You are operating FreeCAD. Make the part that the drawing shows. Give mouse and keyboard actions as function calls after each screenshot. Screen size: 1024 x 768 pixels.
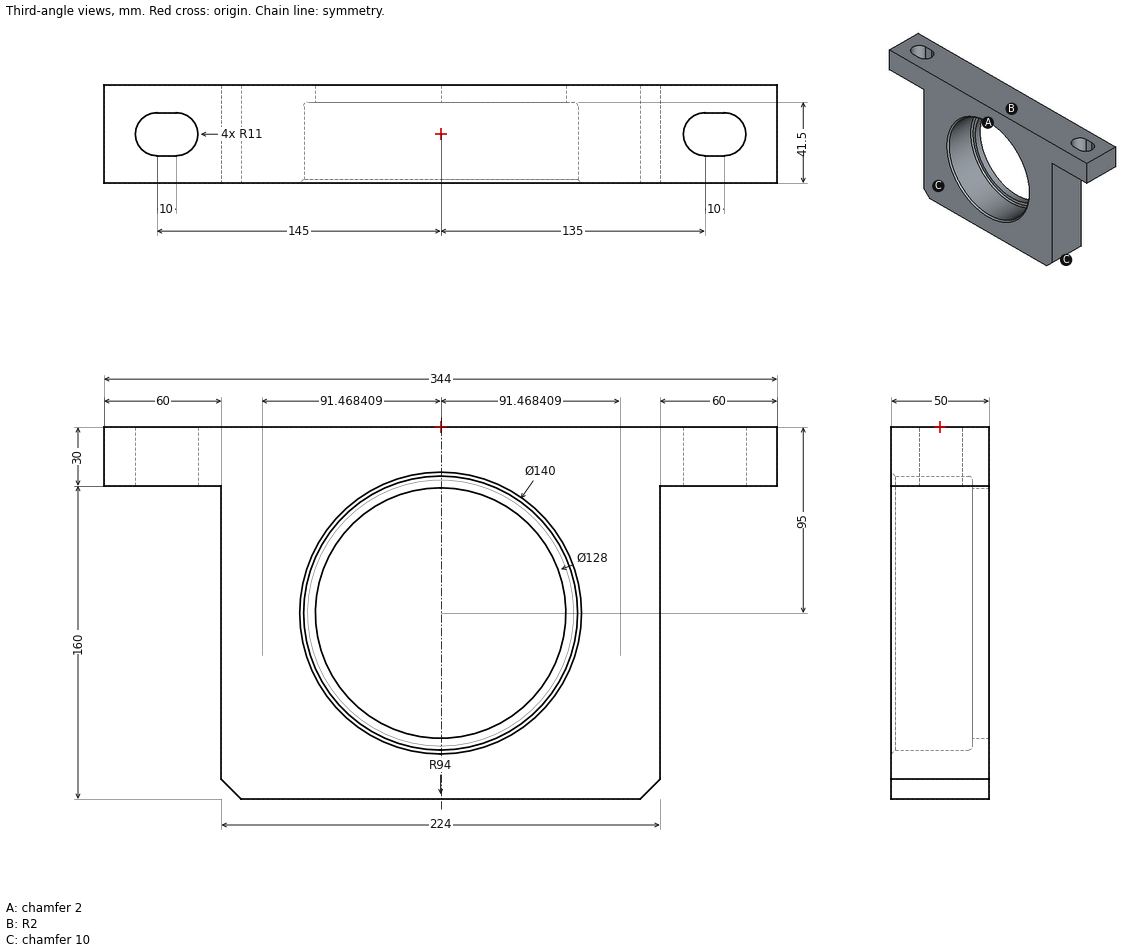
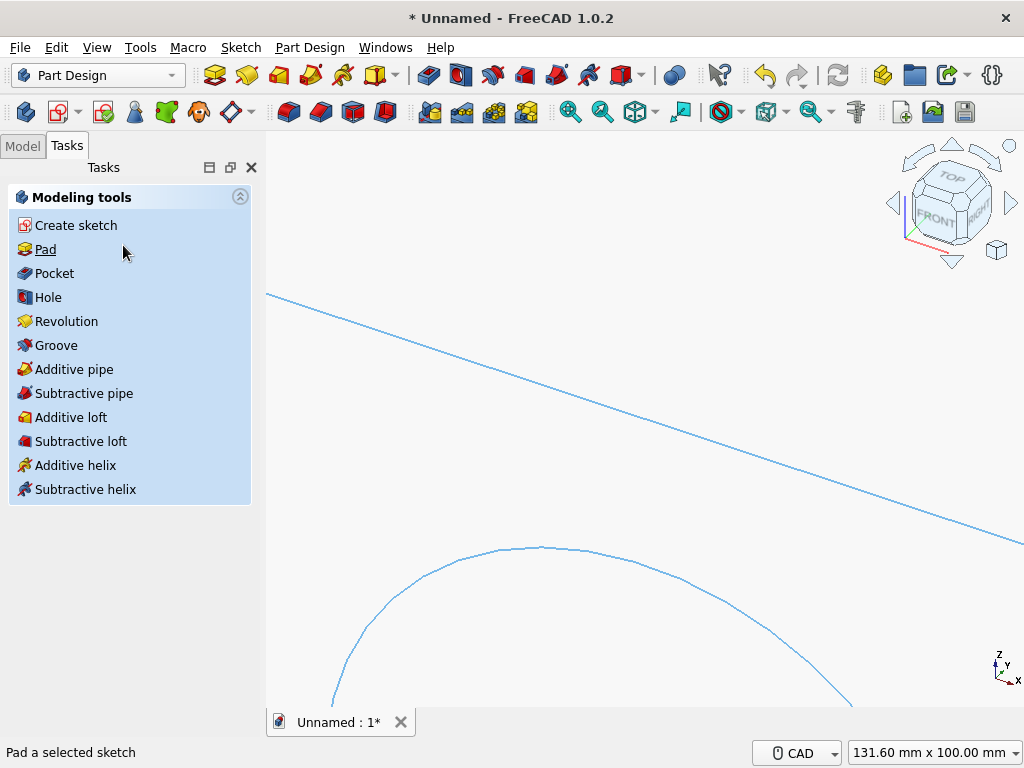
click(216, 76)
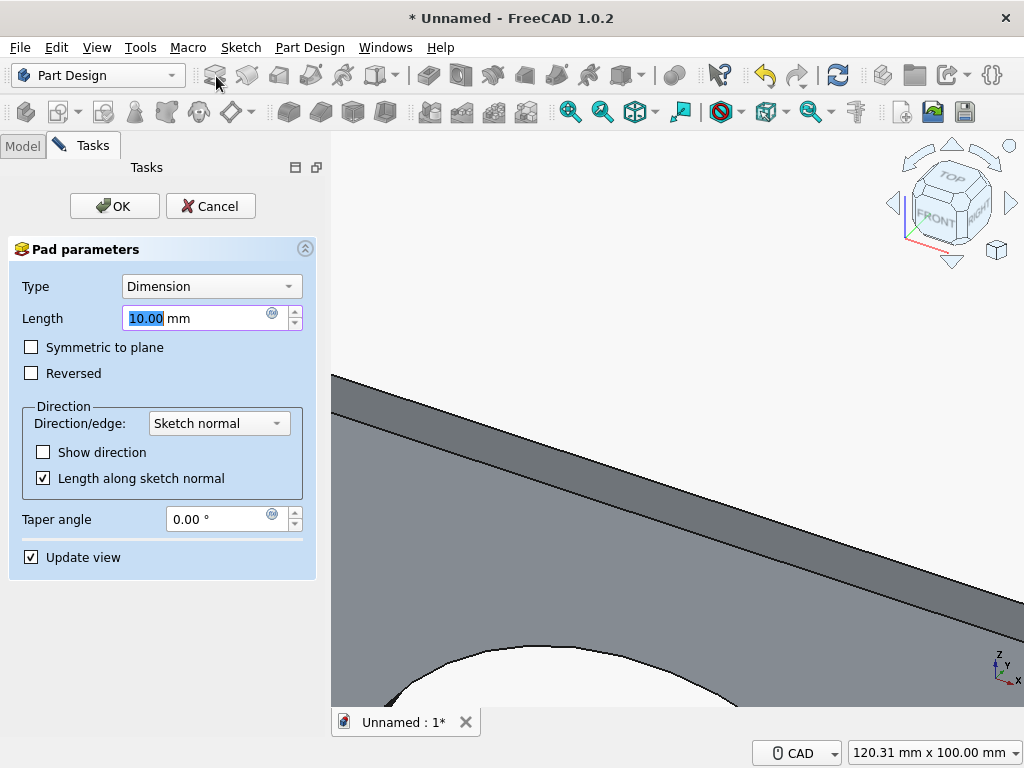
text(50)
key(Tab)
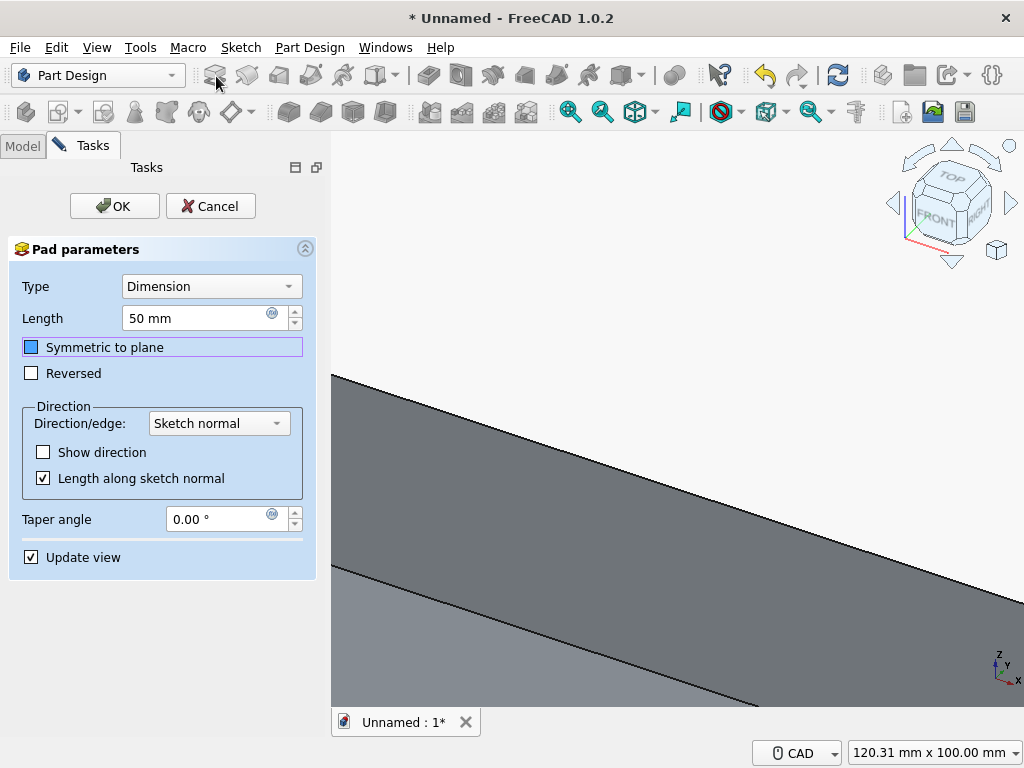
click(30, 347)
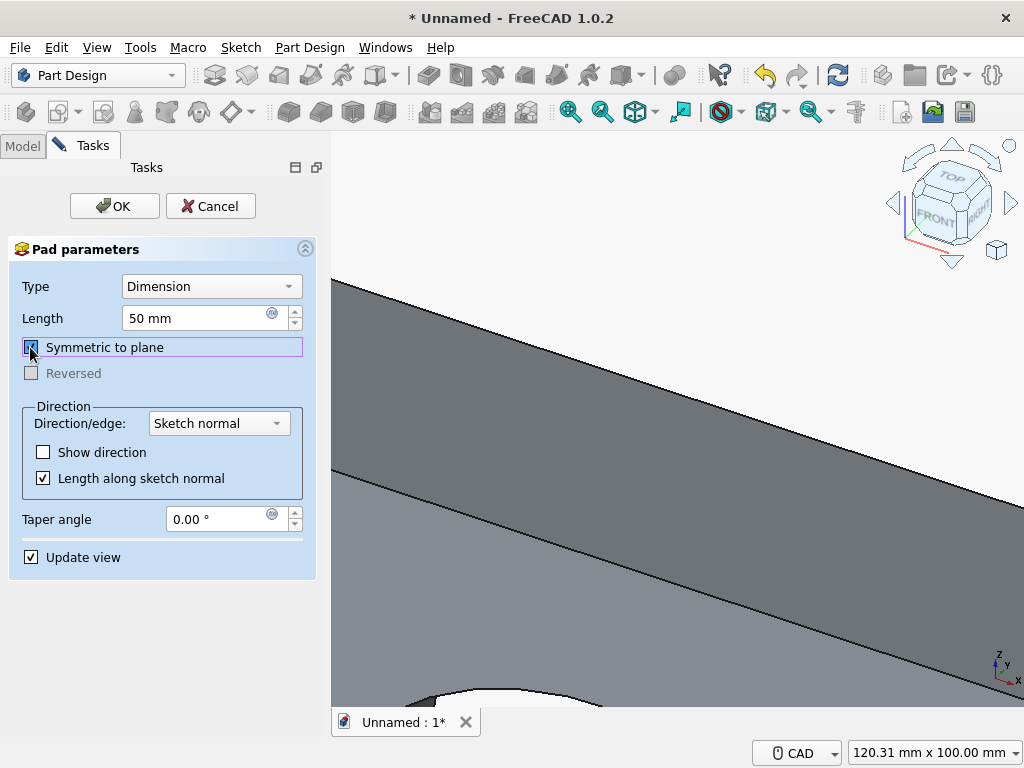
click(115, 206)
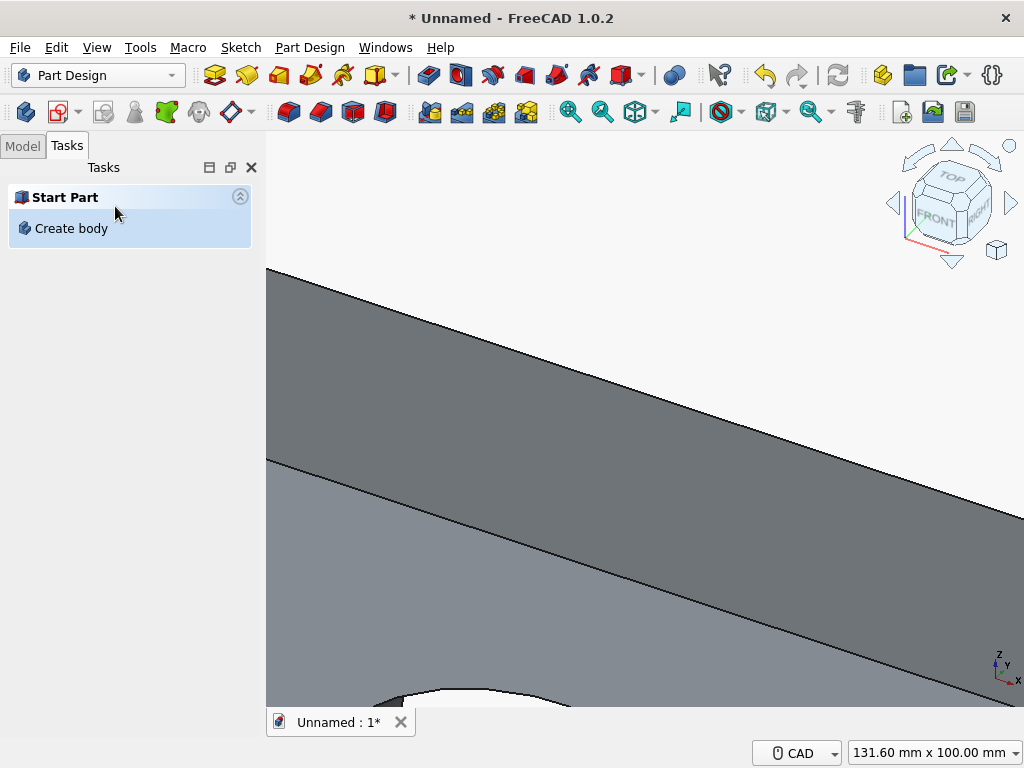
key(v)
key(f)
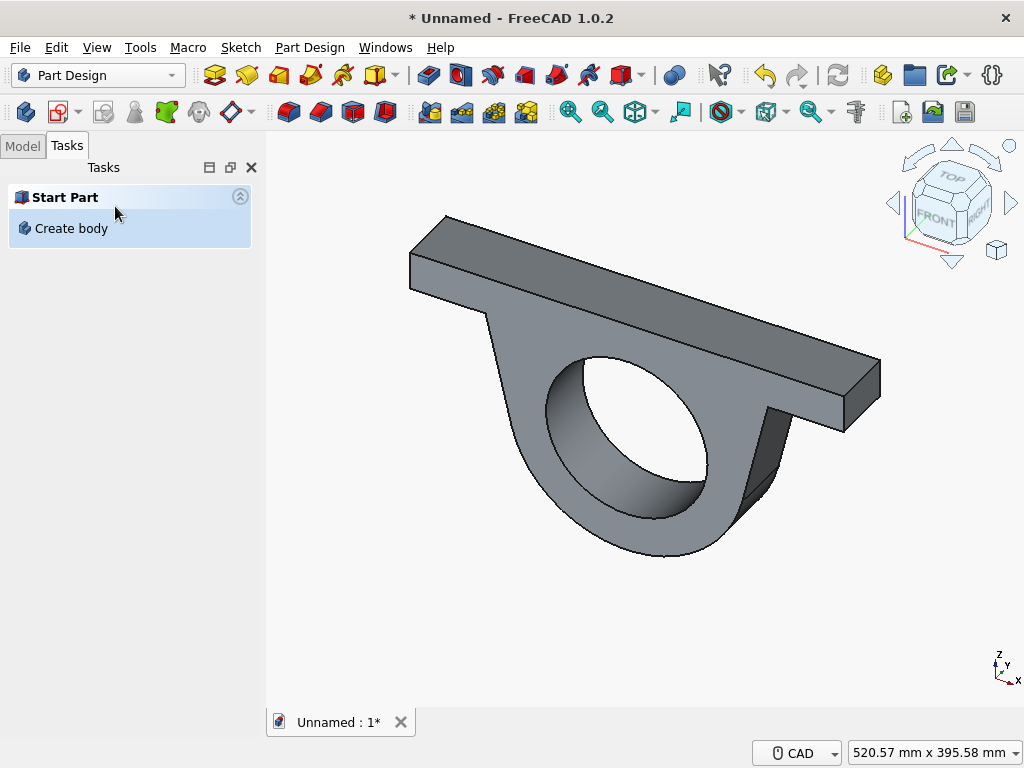
click(813, 401)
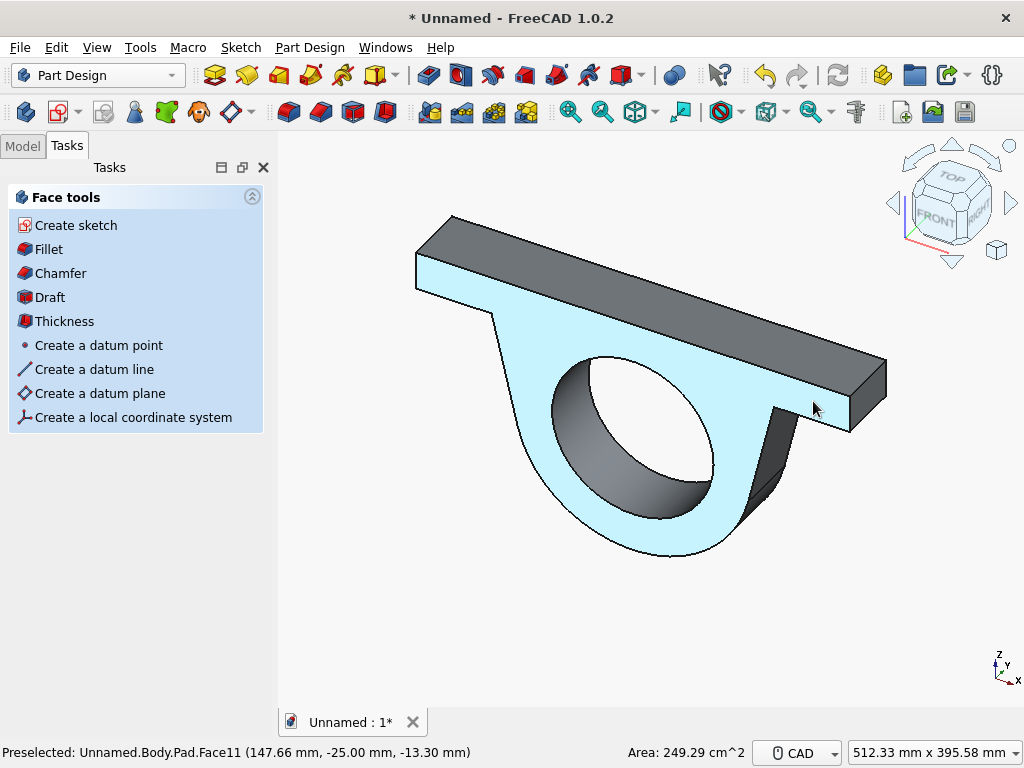
click(58, 112)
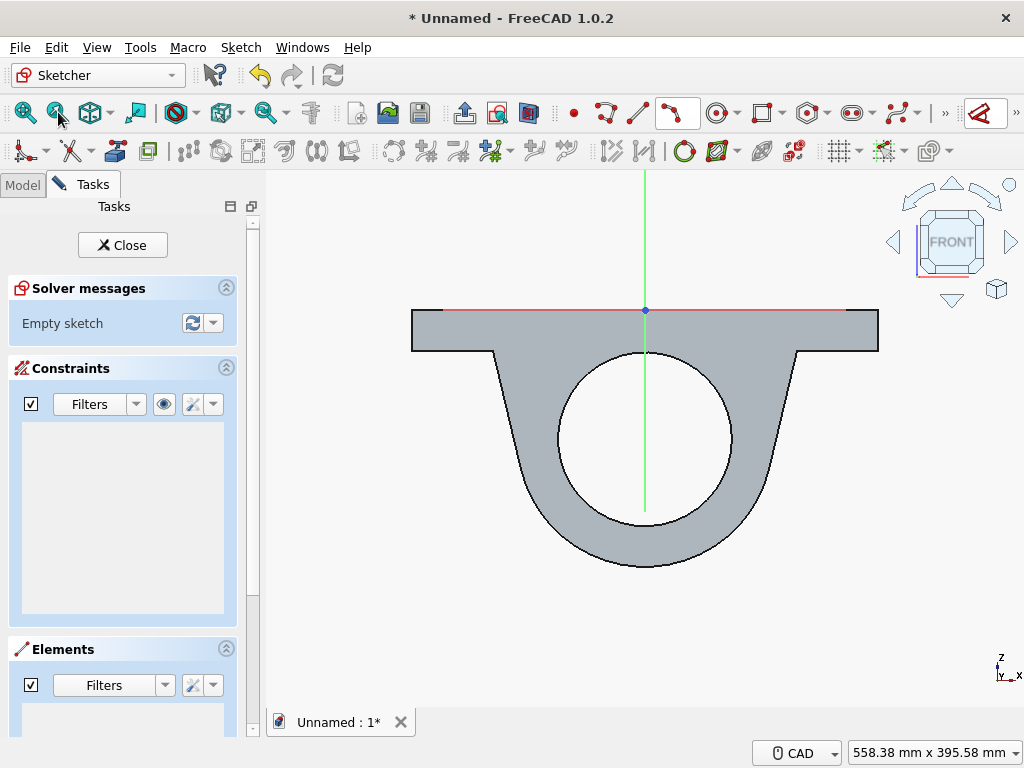
scroll(784, 389, up, 2)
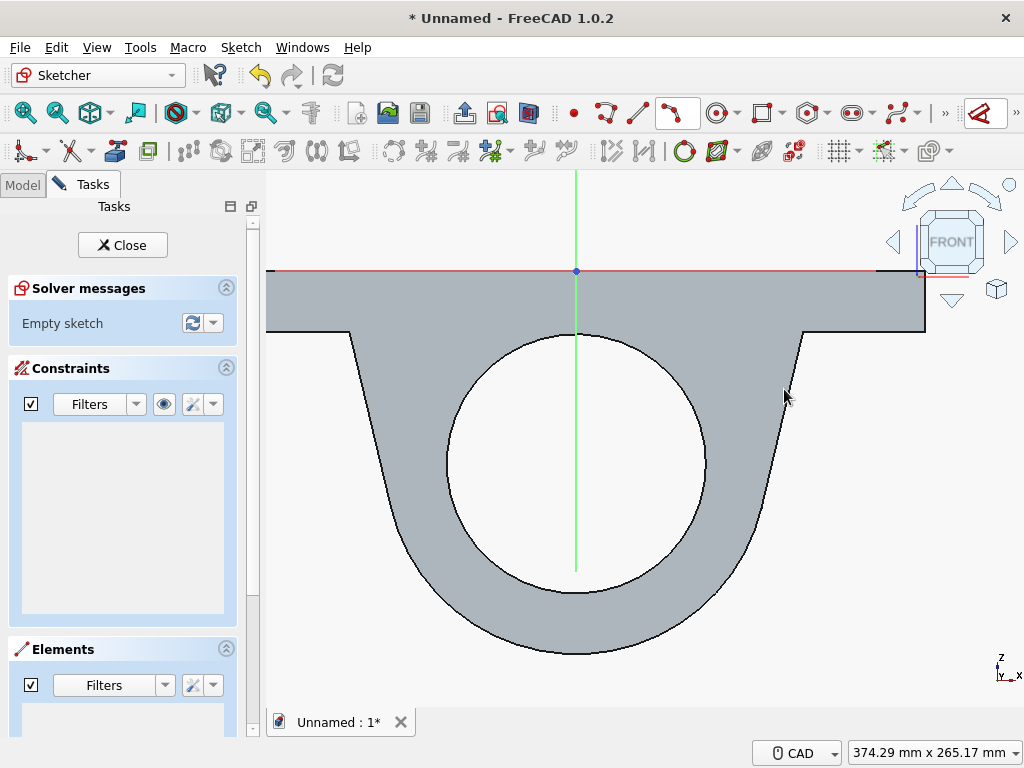
click(718, 114)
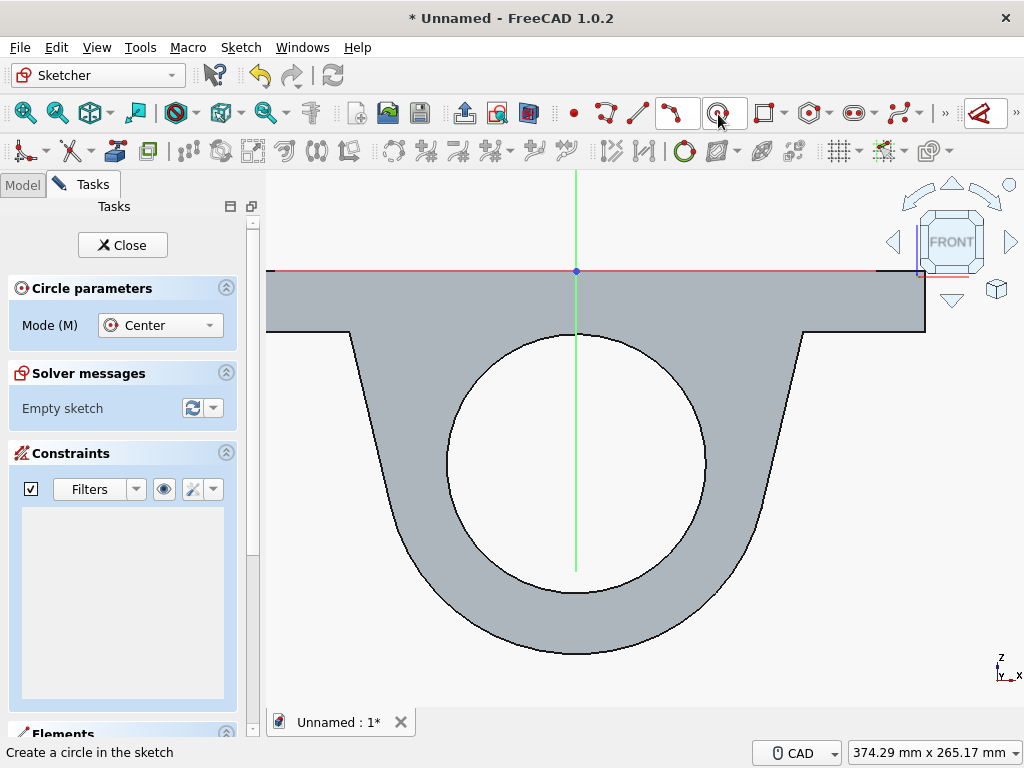
click(576, 464)
move(677, 364)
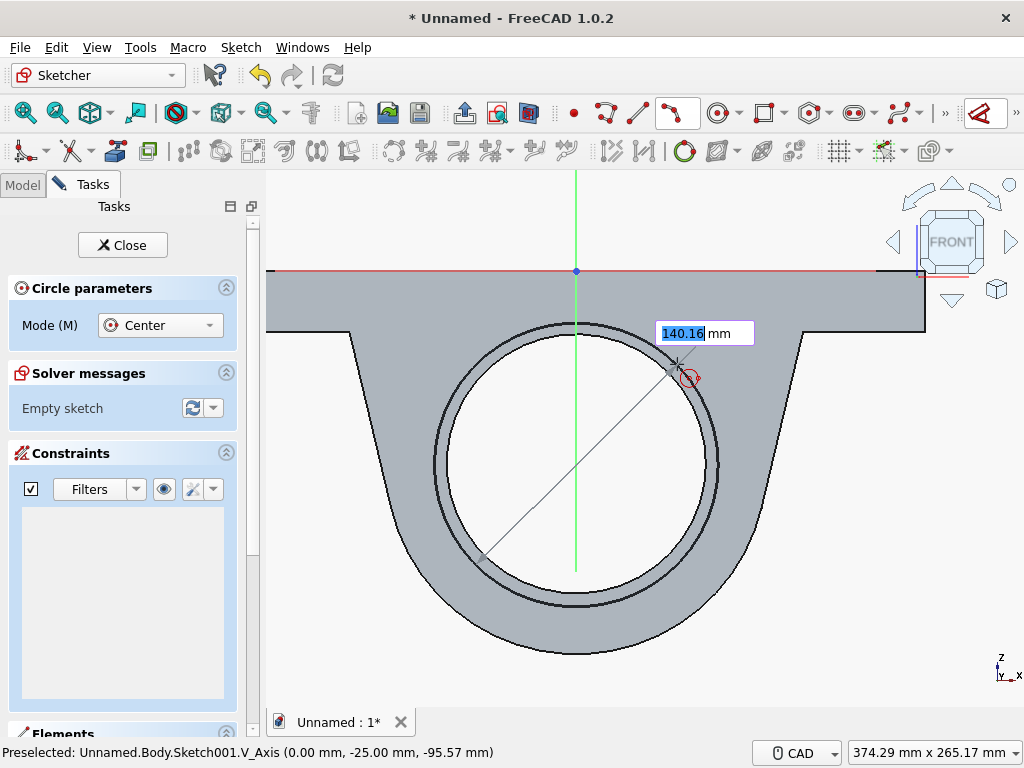
text(140)
key(Return)
key(Escape)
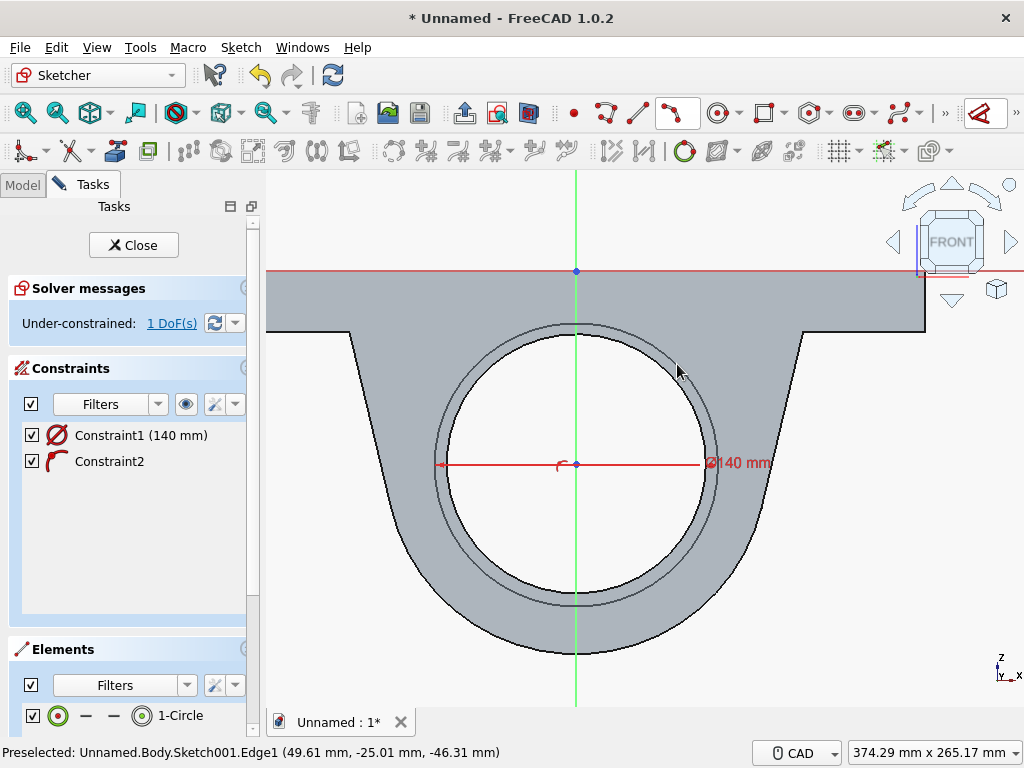
key(d)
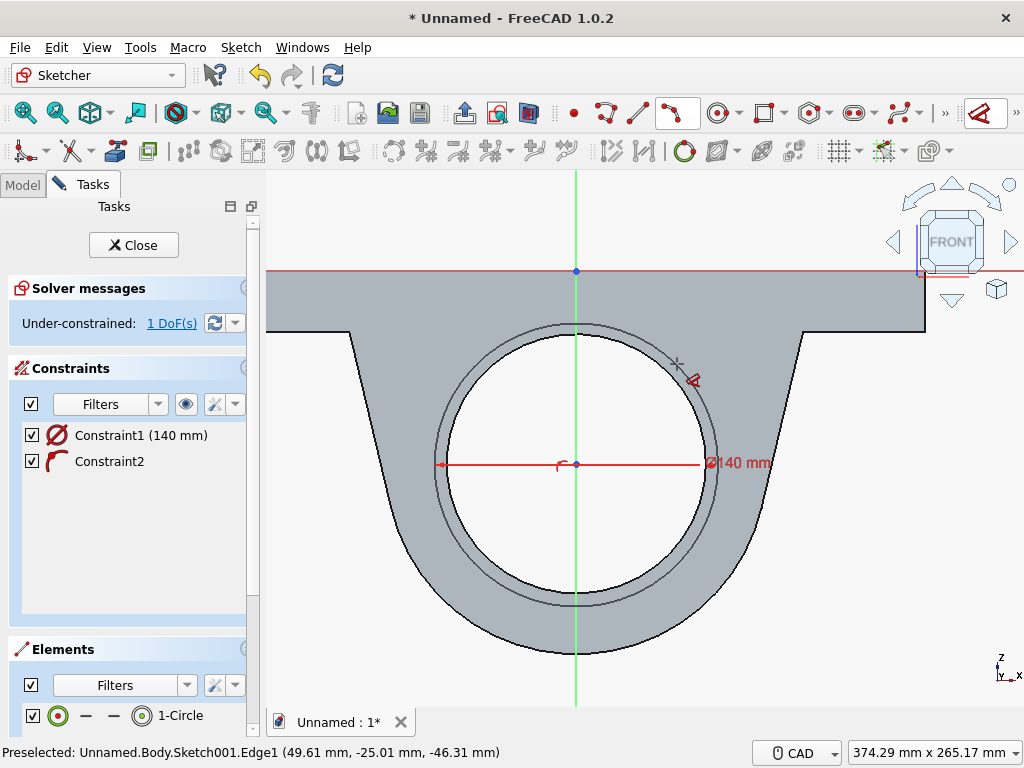
click(576, 465)
click(610, 368)